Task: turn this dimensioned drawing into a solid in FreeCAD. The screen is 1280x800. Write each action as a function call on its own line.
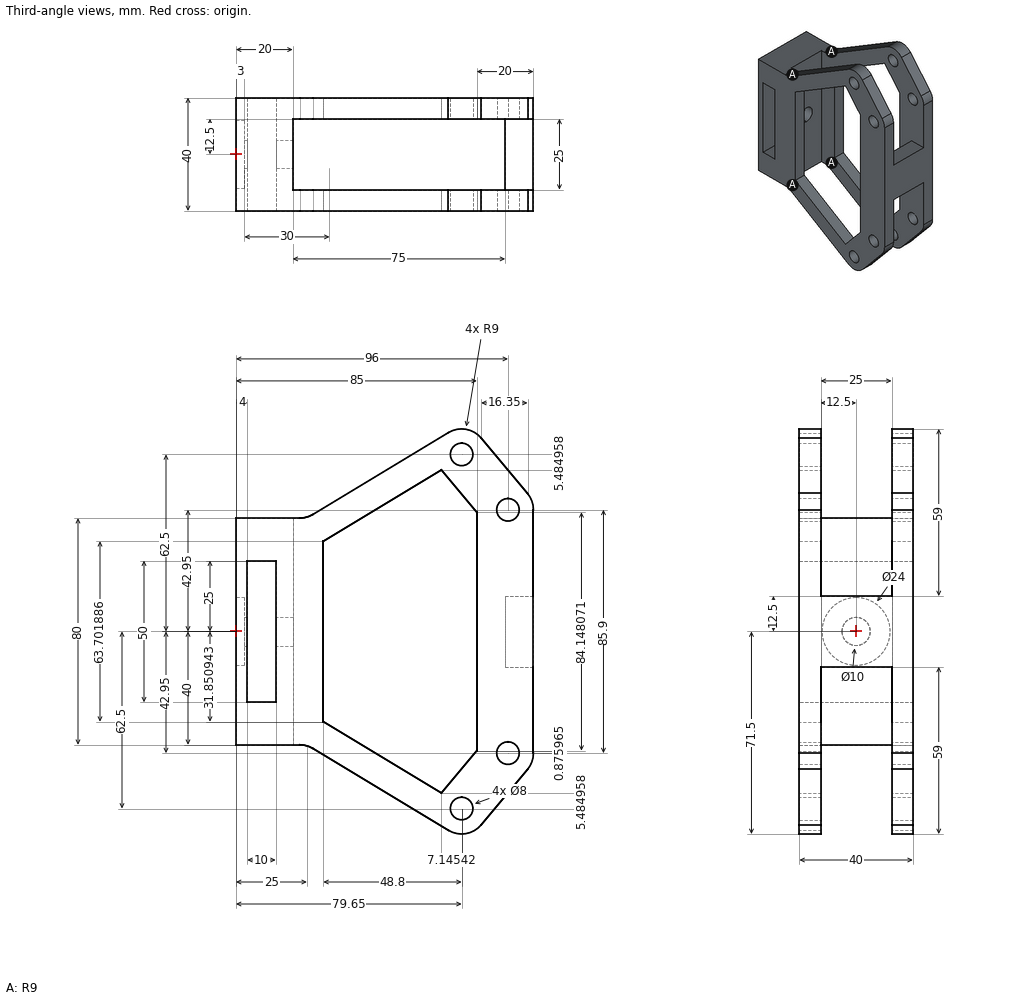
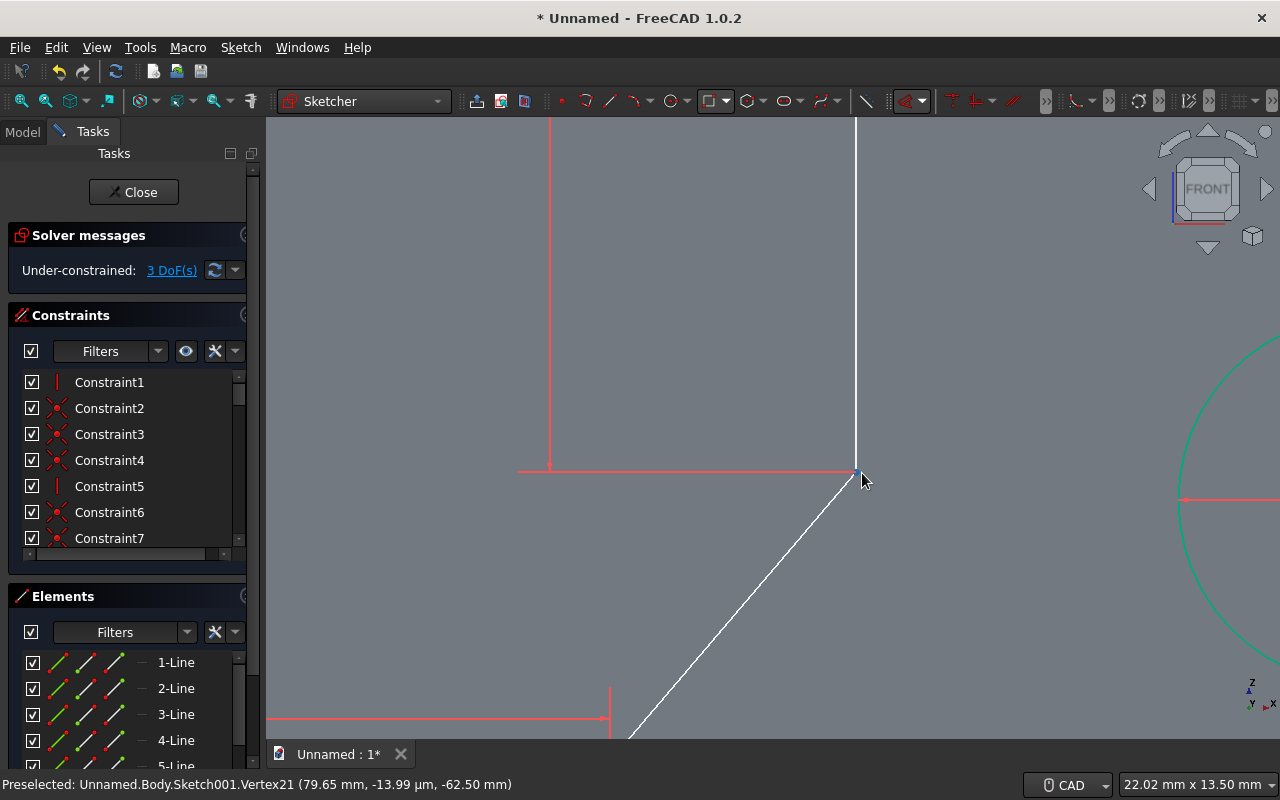
click(856, 472)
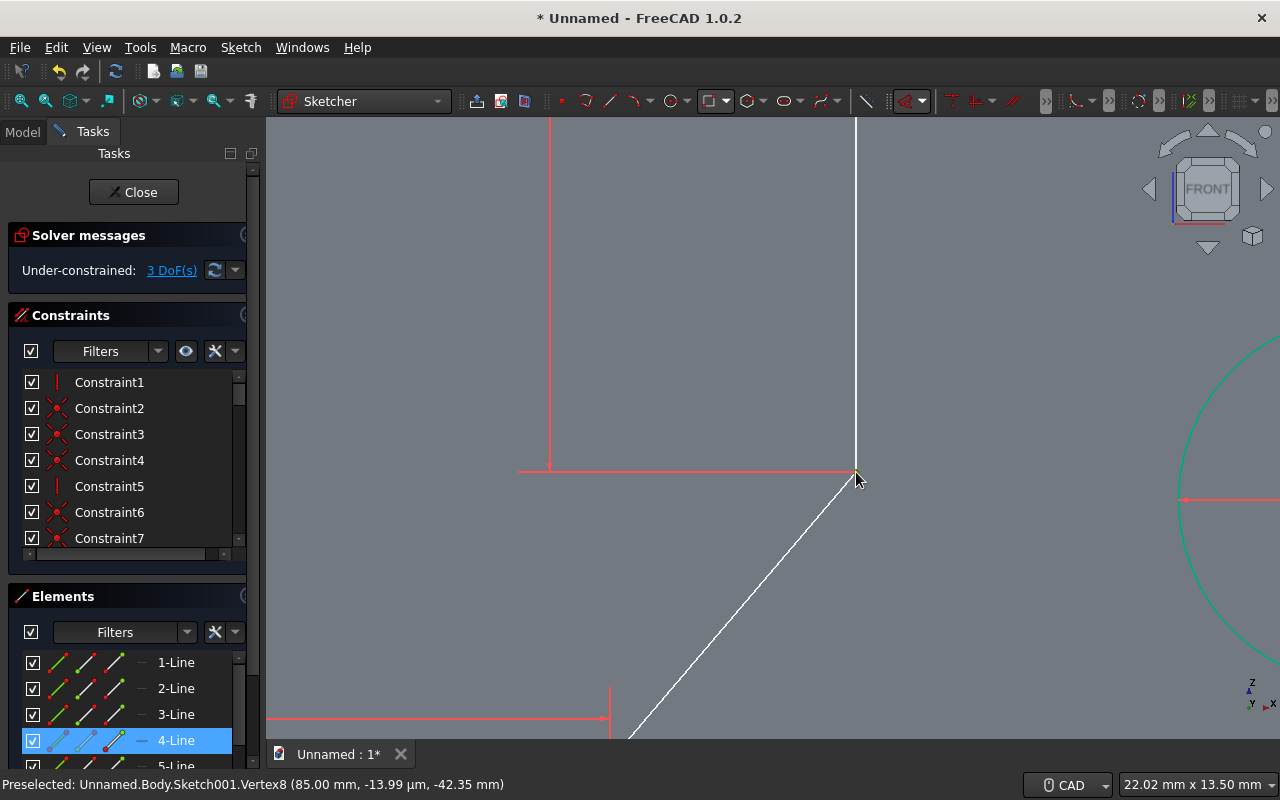
scroll(799, 551, down, 14)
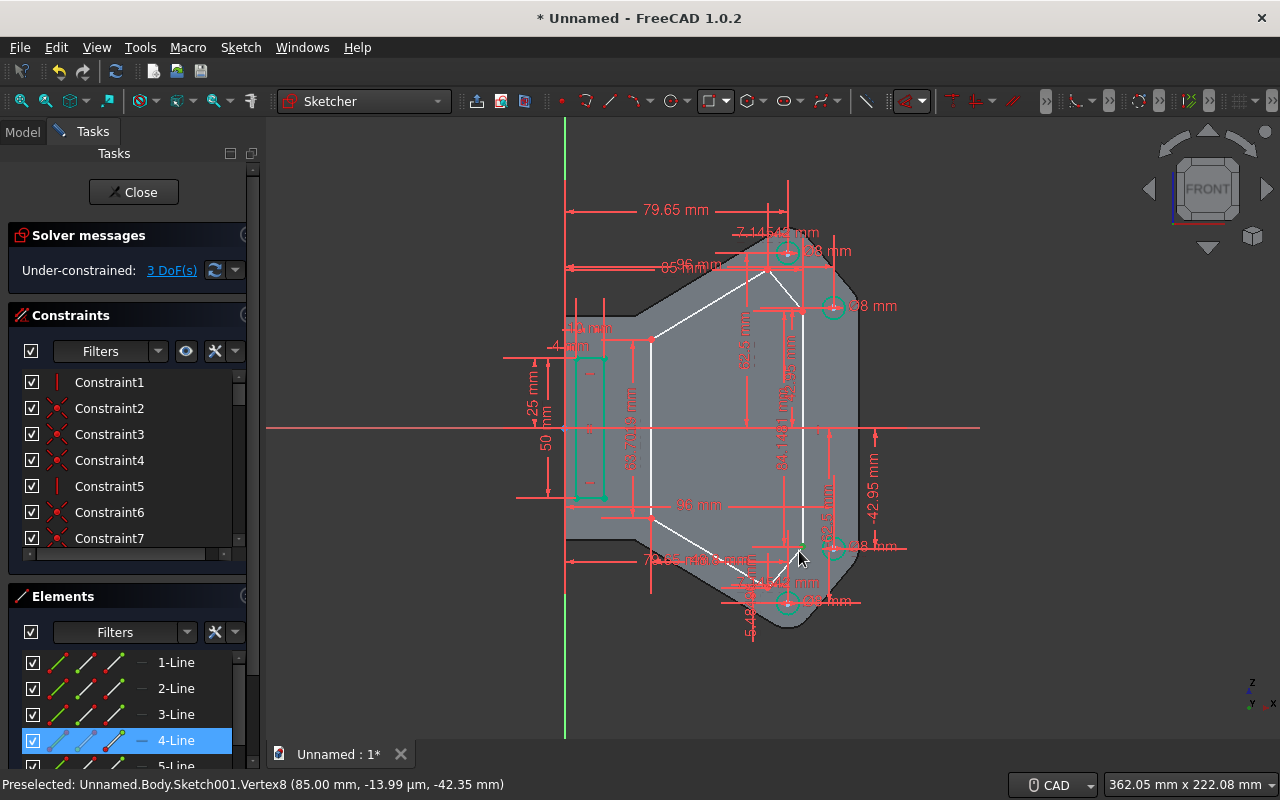
scroll(834, 549, up, 14)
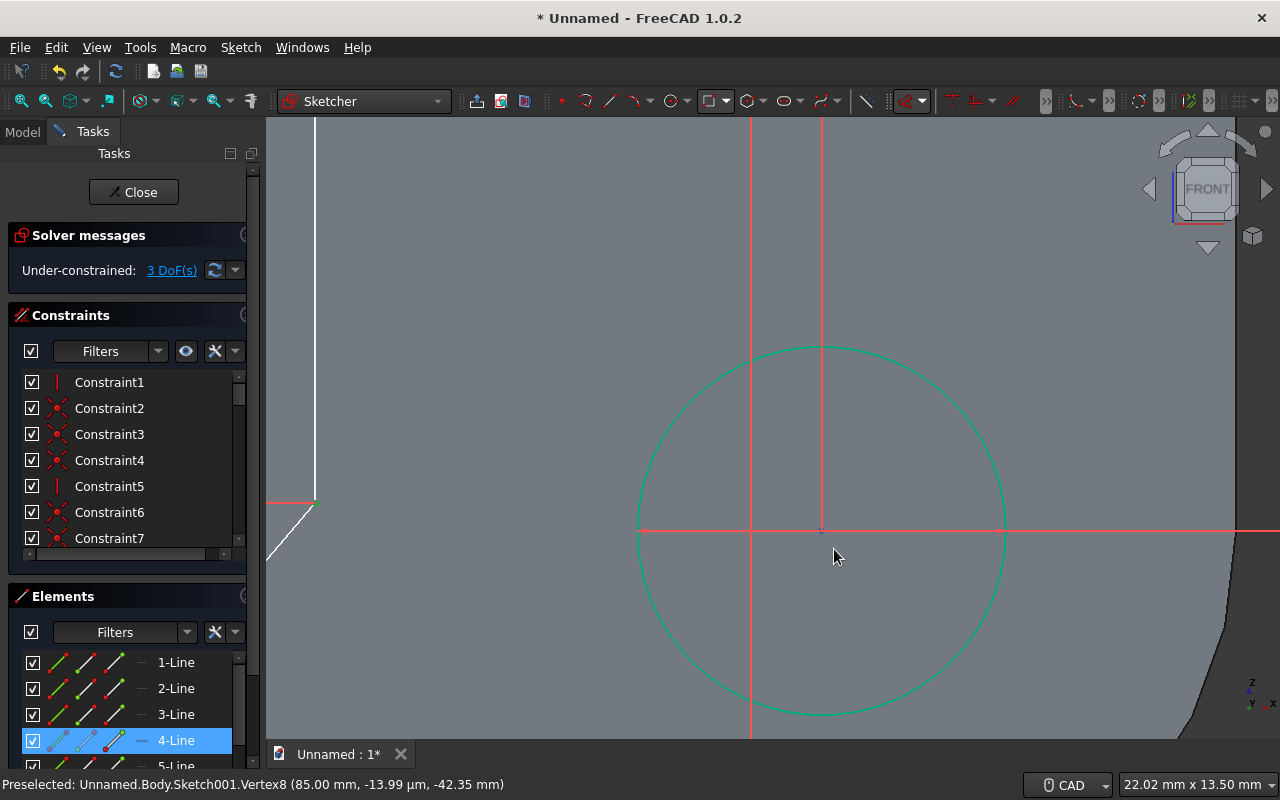
click(822, 531)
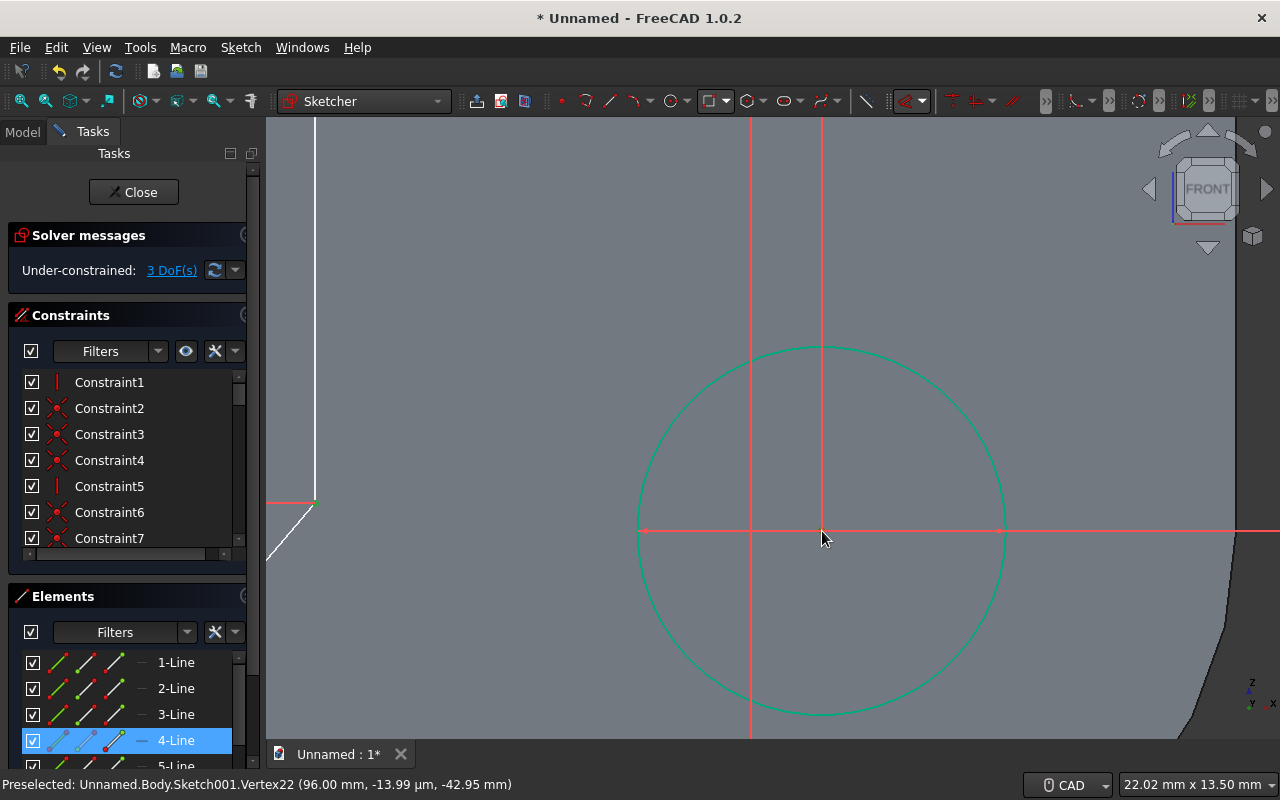
key(i)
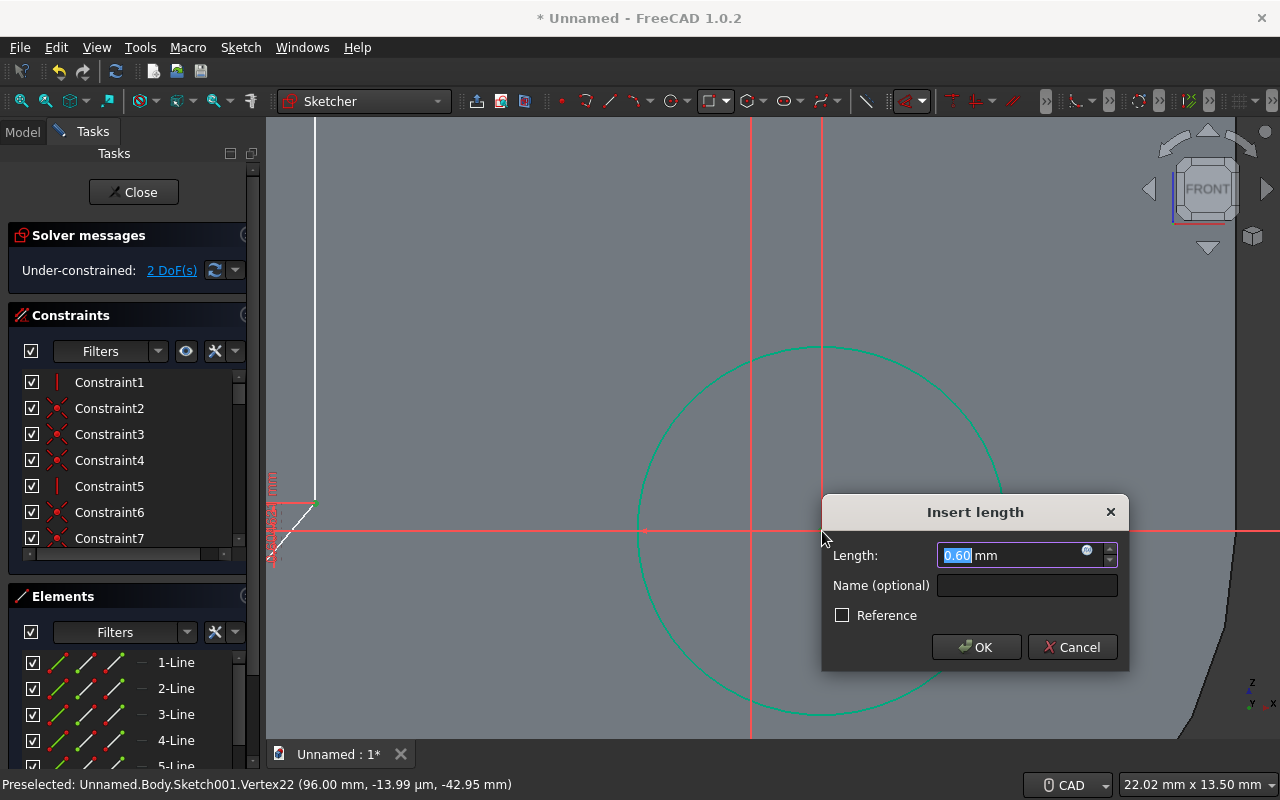
text(0.875965)
key(Return)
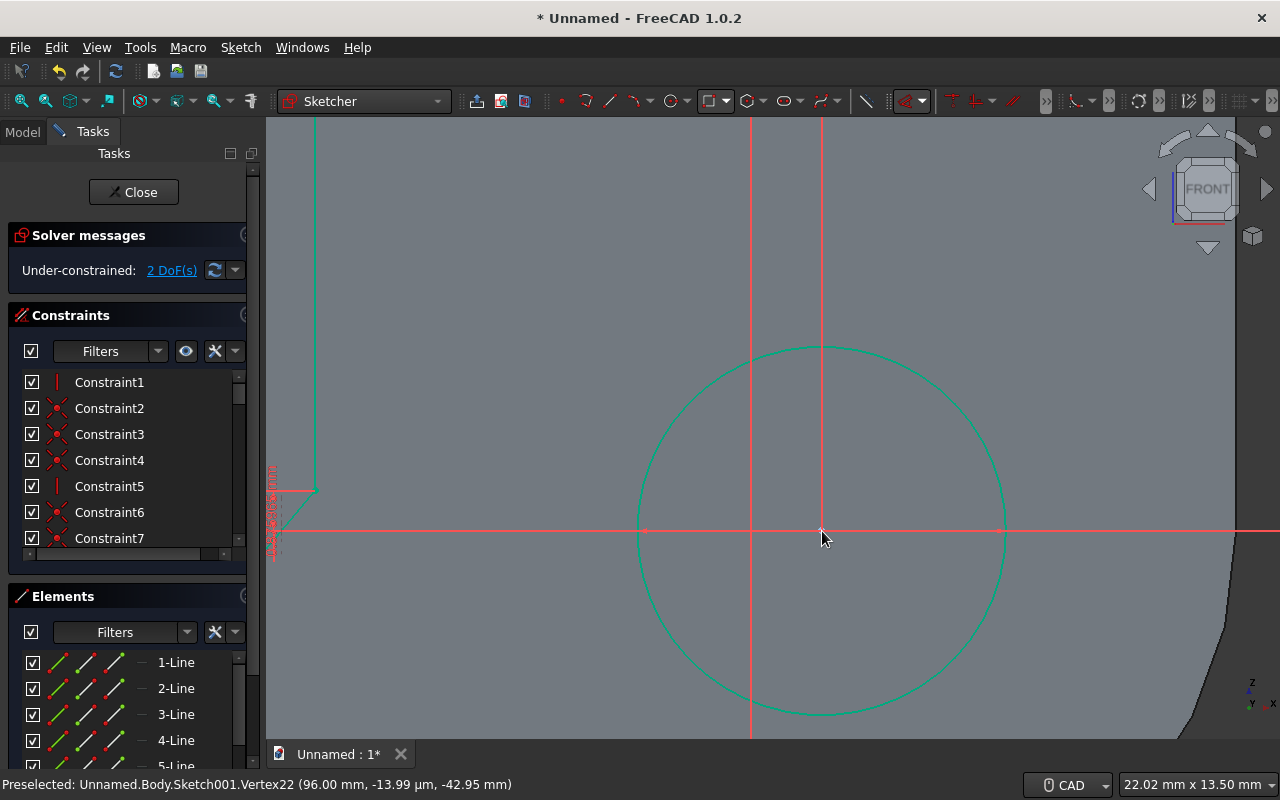
scroll(834, 549, down, 14)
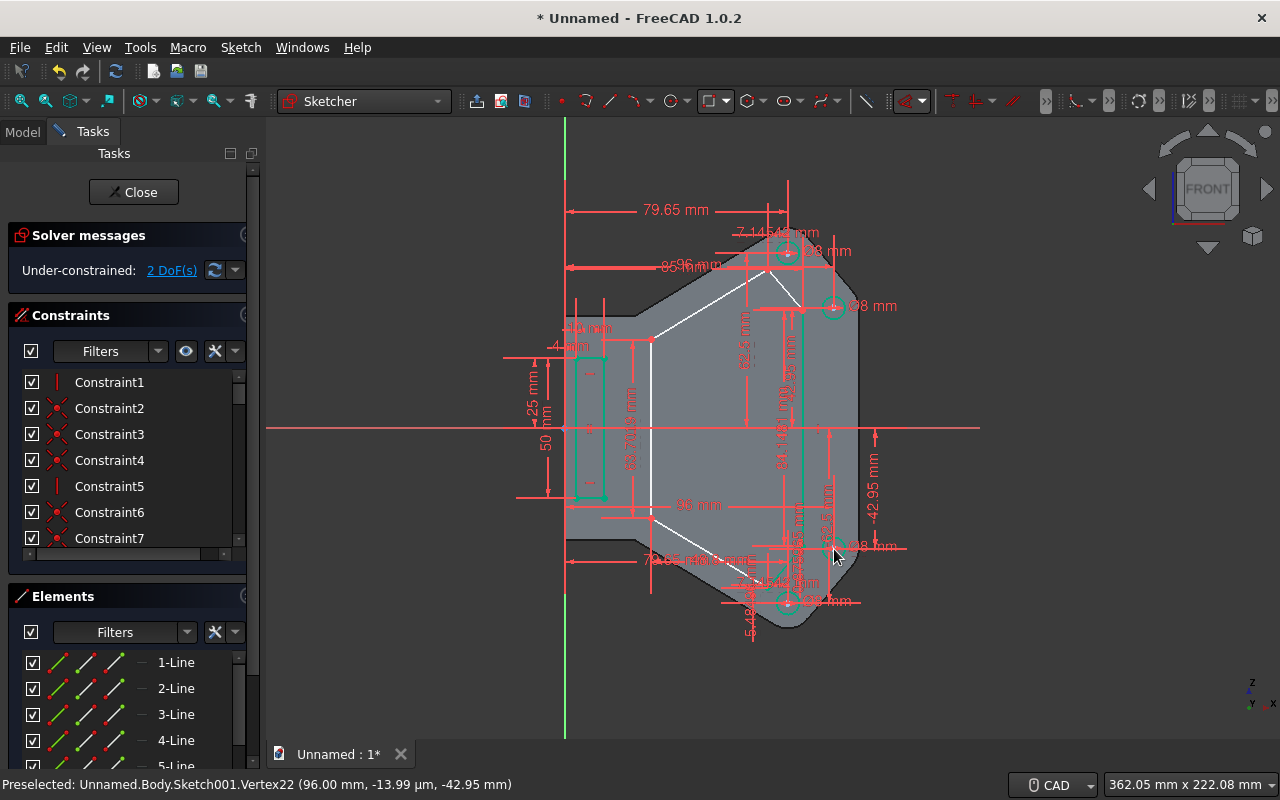
scroll(768, 269, up, 5)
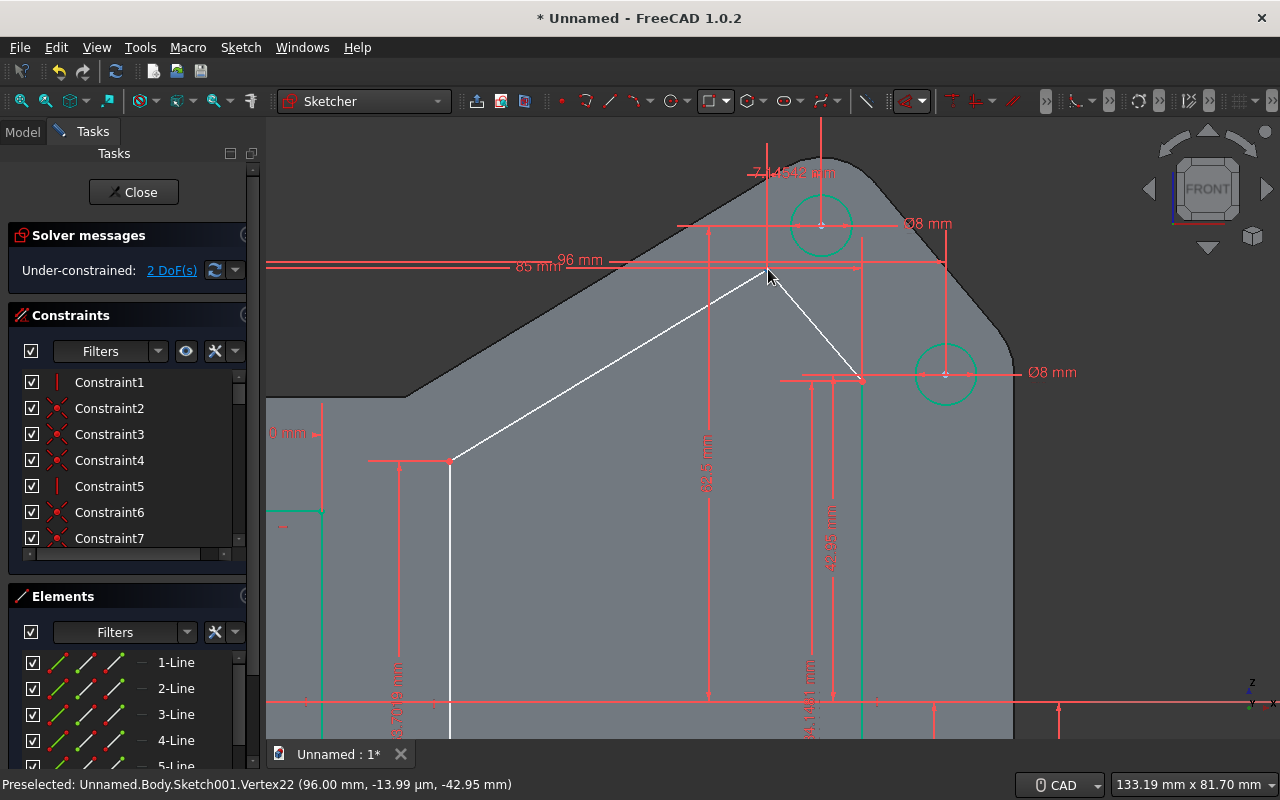
click(767, 270)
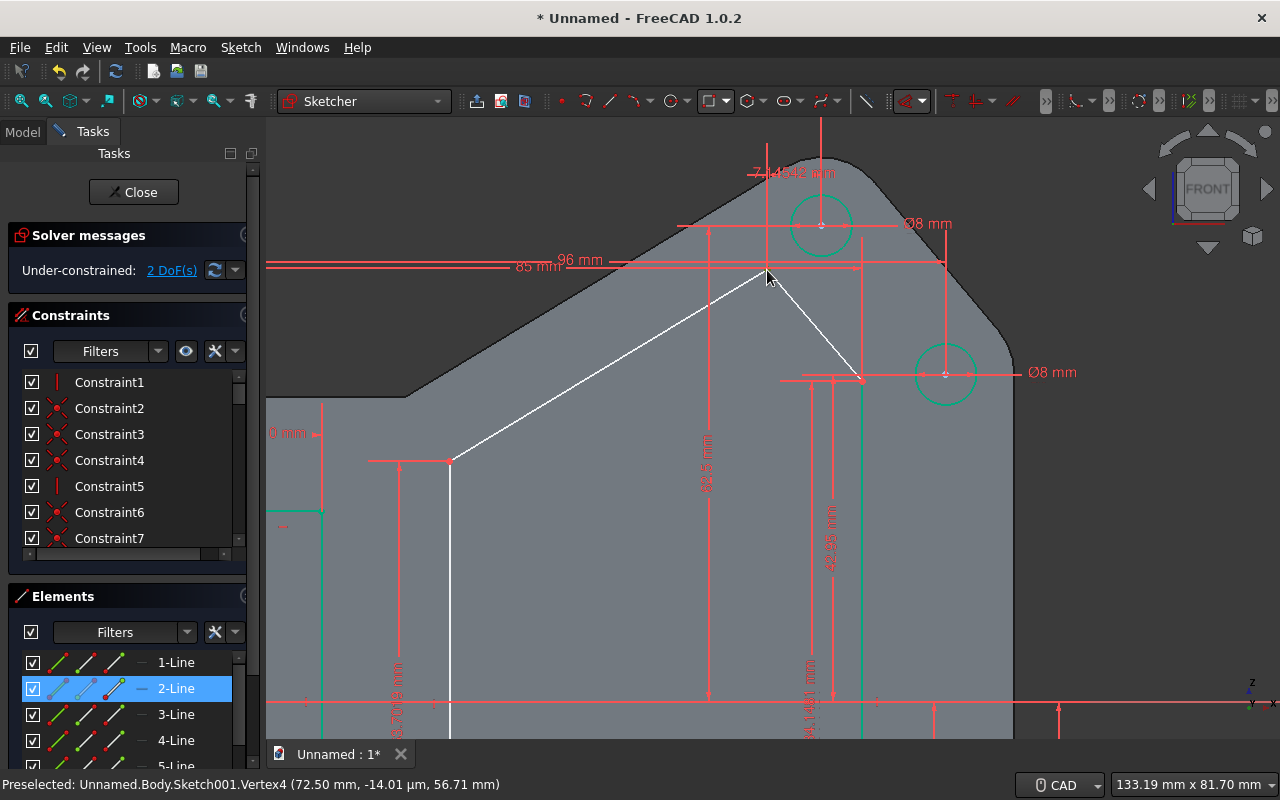
click(821, 226)